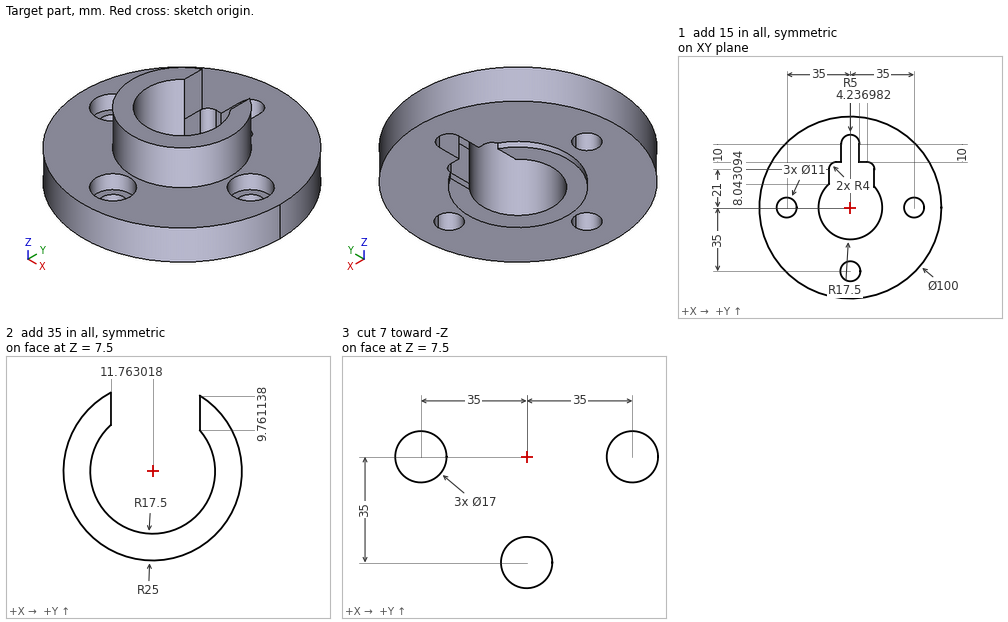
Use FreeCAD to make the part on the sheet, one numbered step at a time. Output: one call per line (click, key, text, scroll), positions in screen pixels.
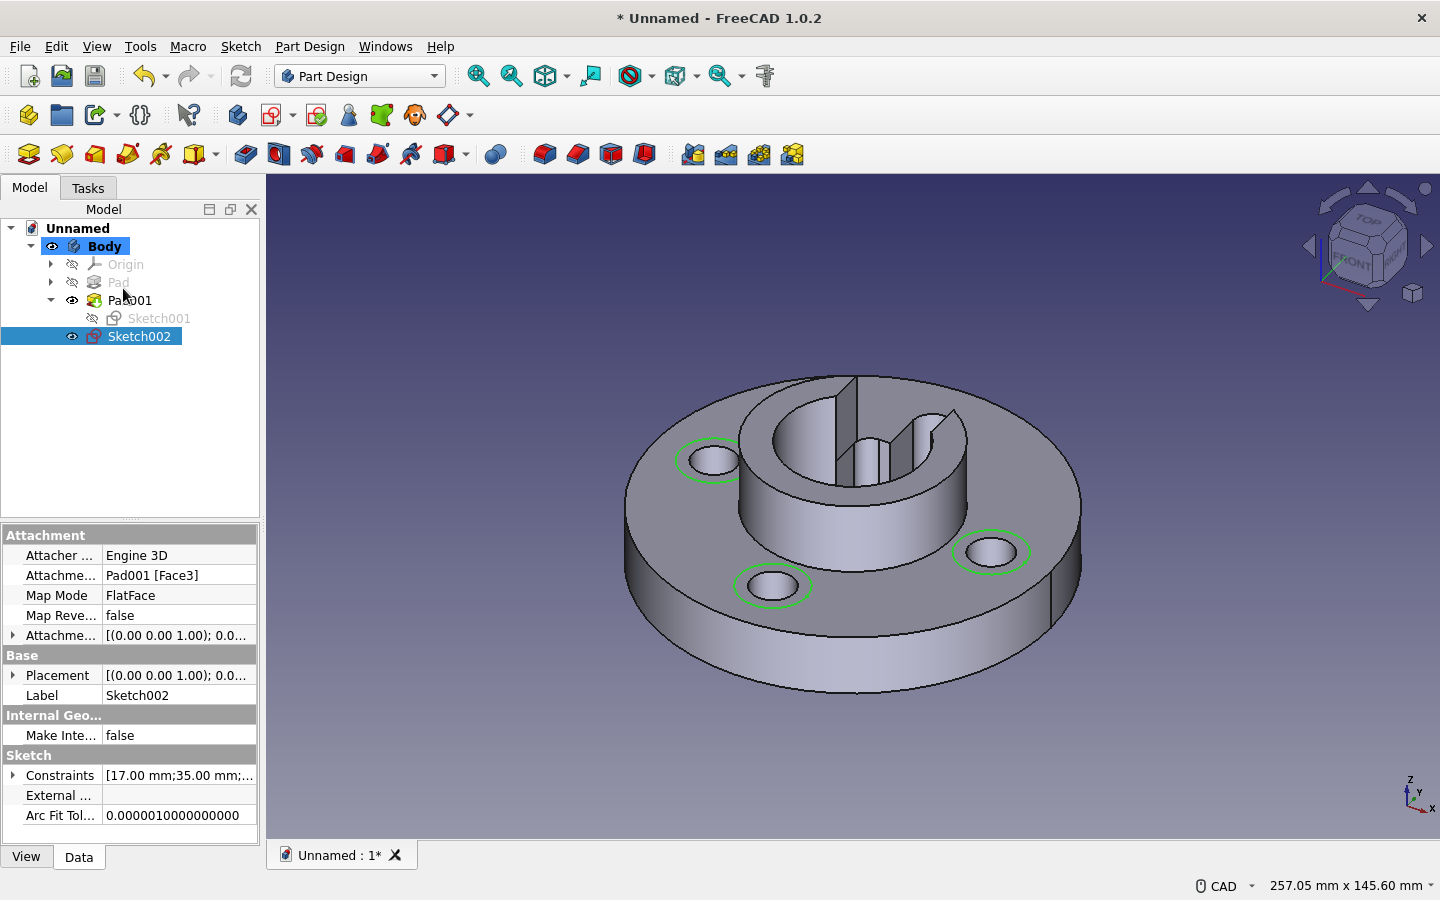
click(246, 154)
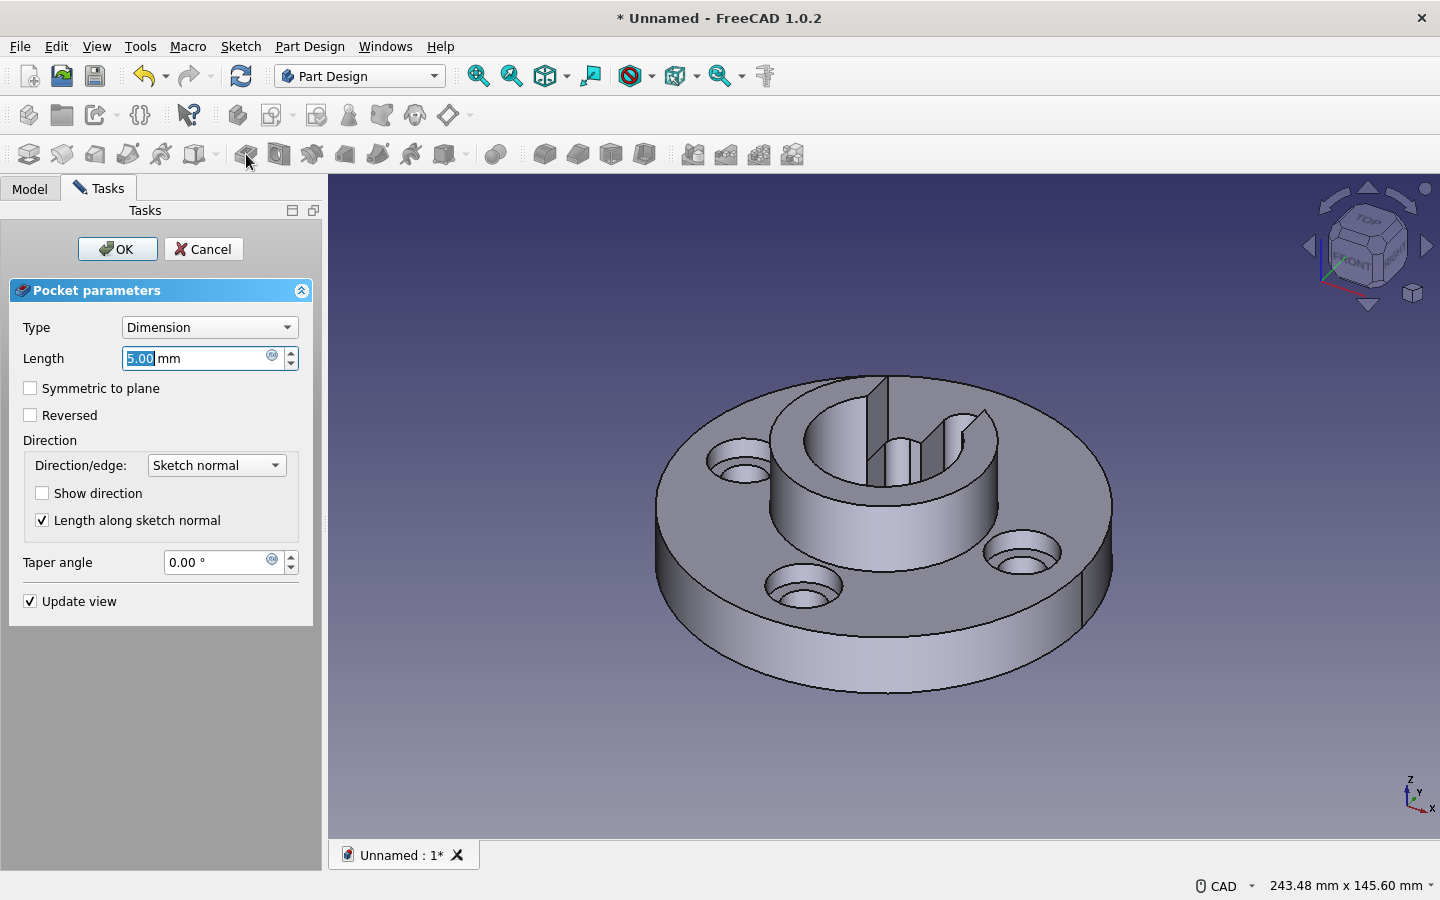
text(7)
key(Tab)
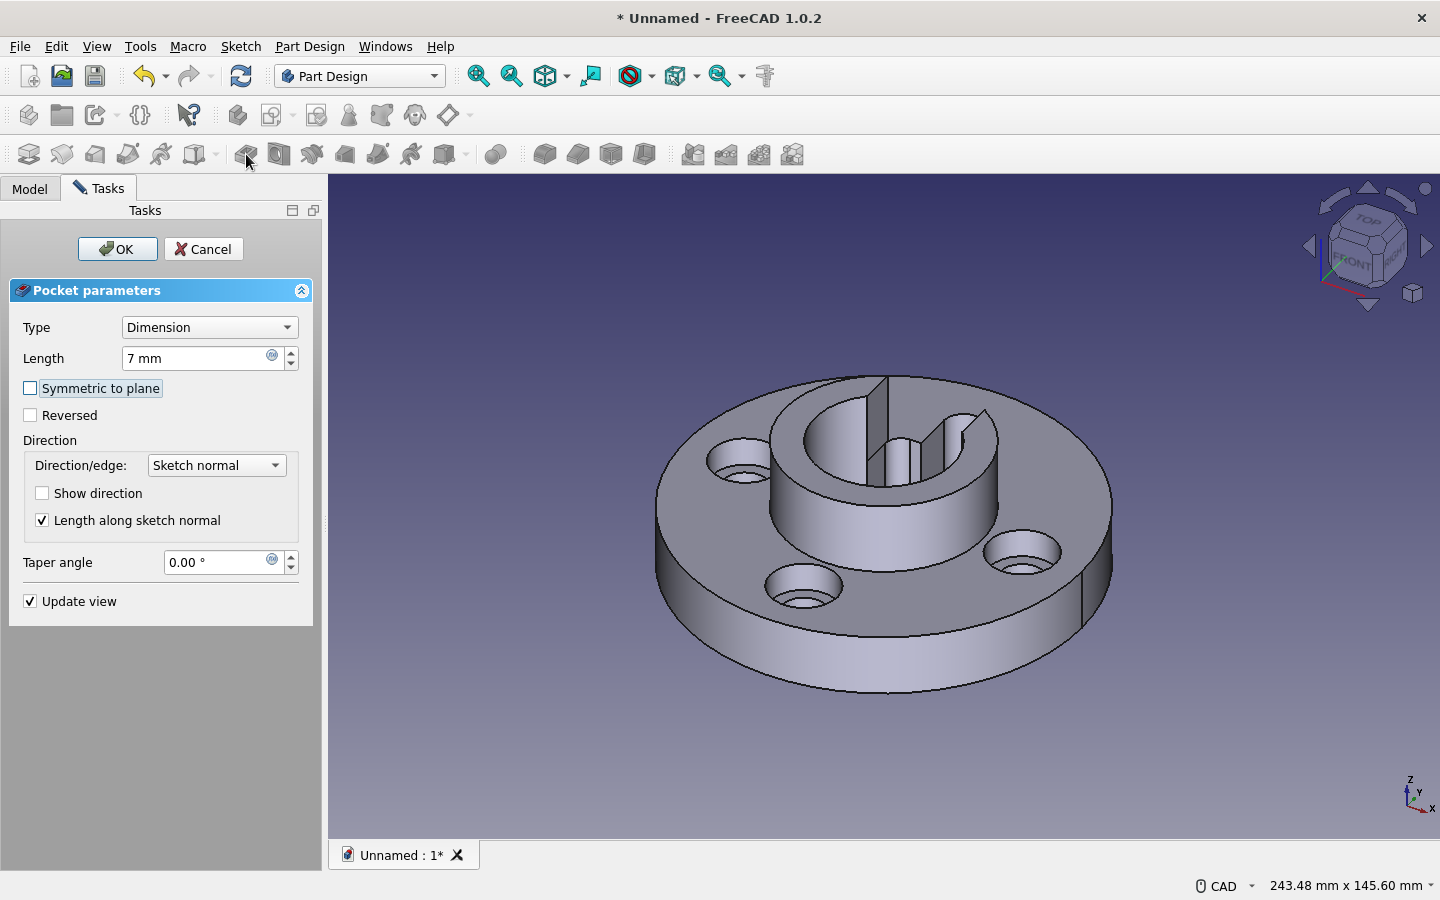
click(118, 249)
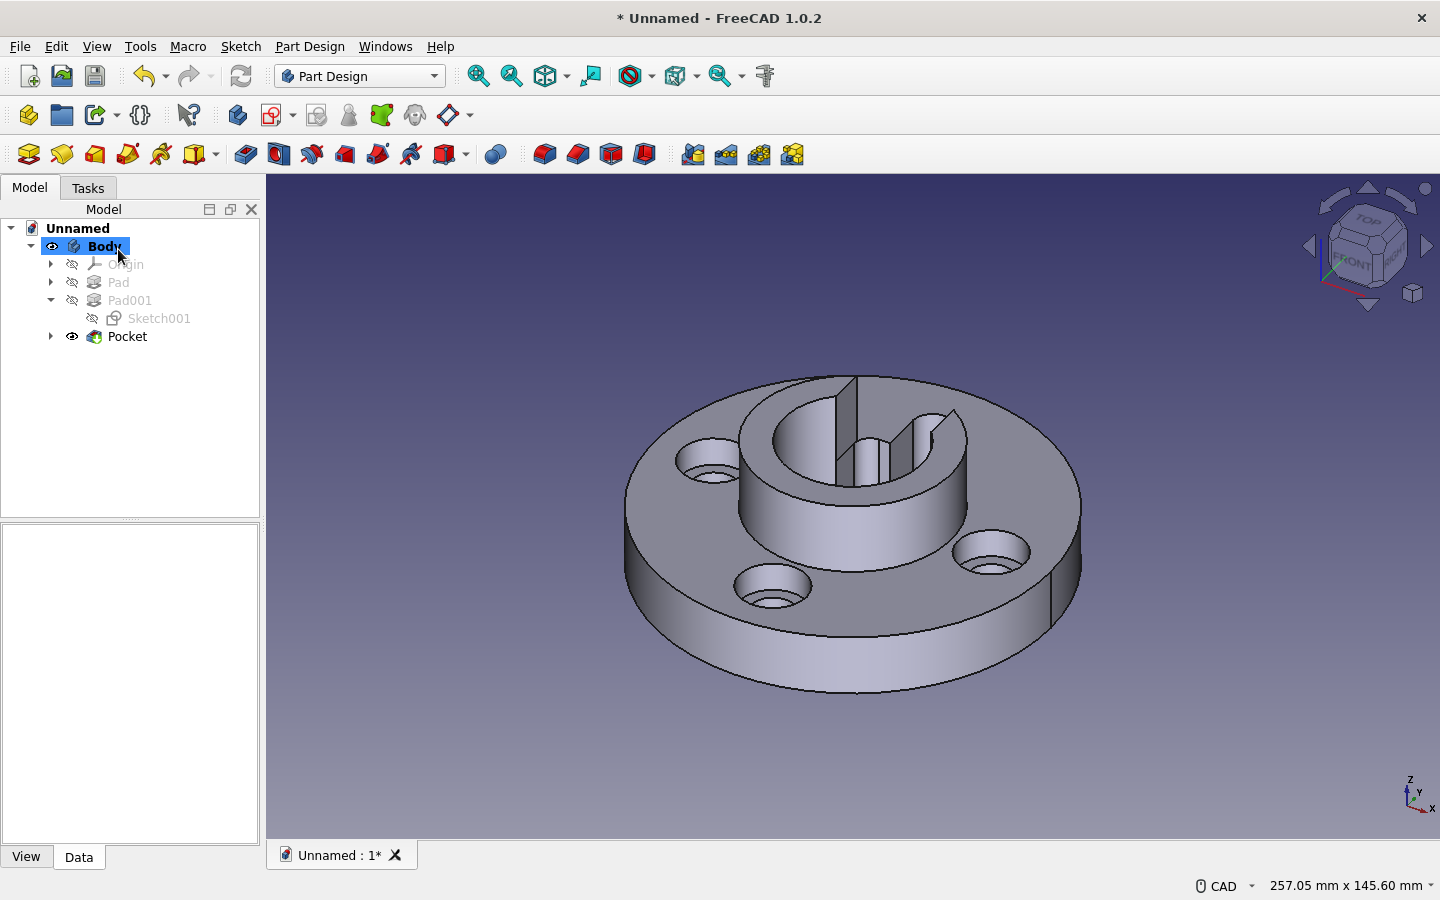
key(0)